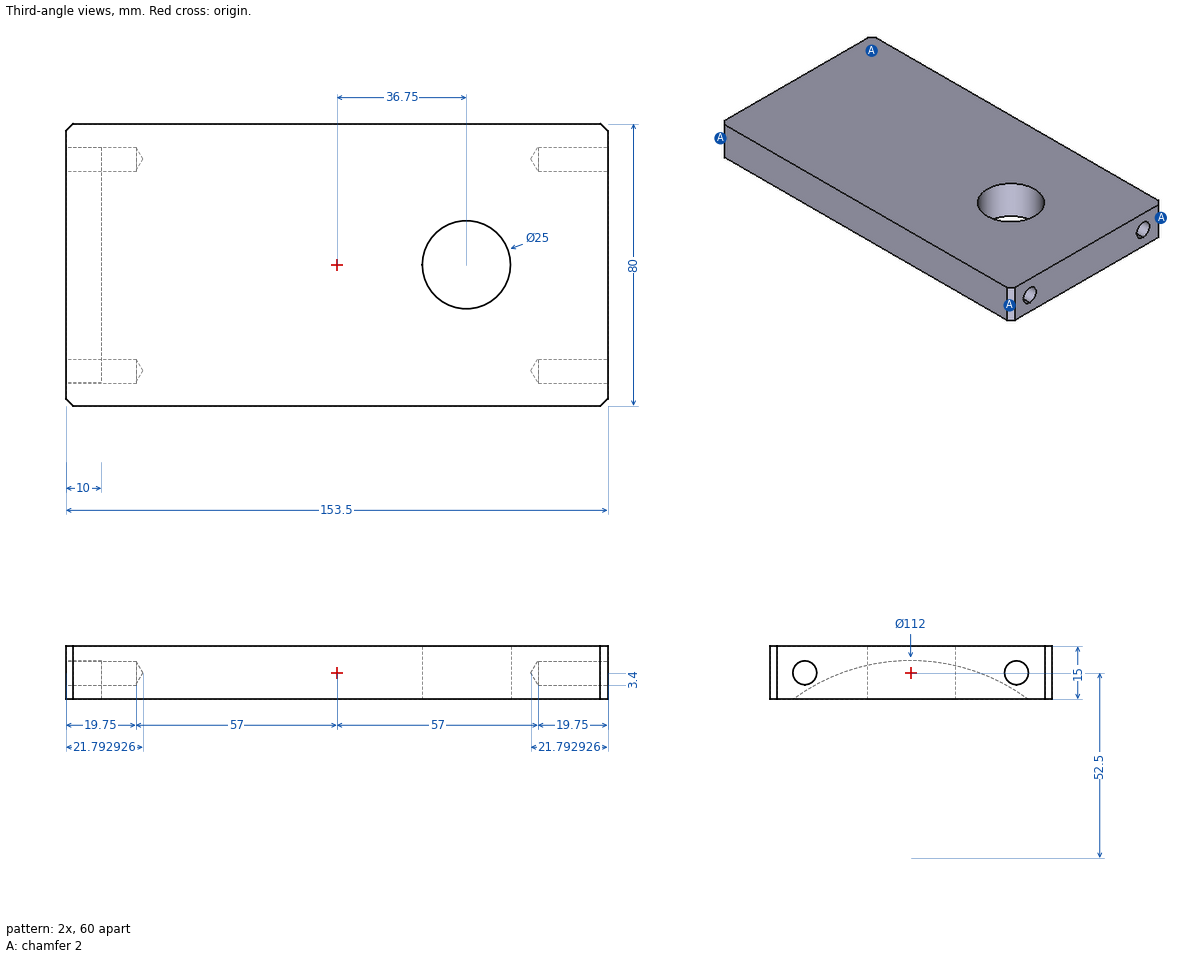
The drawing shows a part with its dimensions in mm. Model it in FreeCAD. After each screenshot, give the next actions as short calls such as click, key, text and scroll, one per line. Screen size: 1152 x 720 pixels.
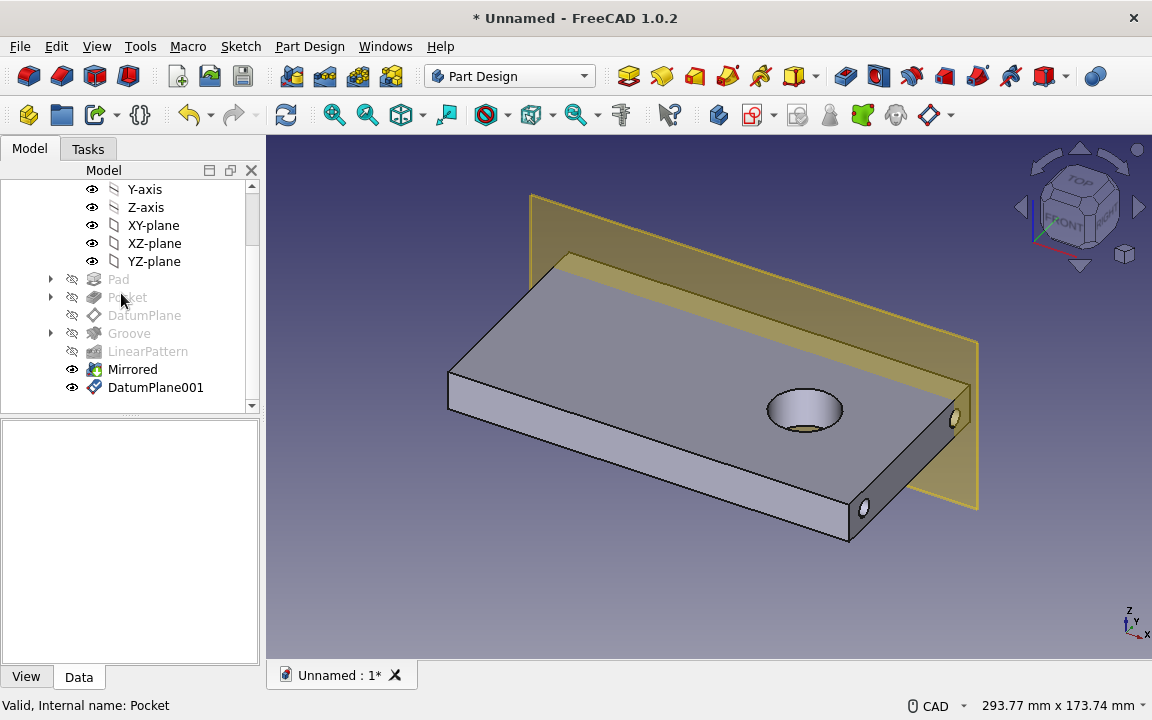
click(117, 387)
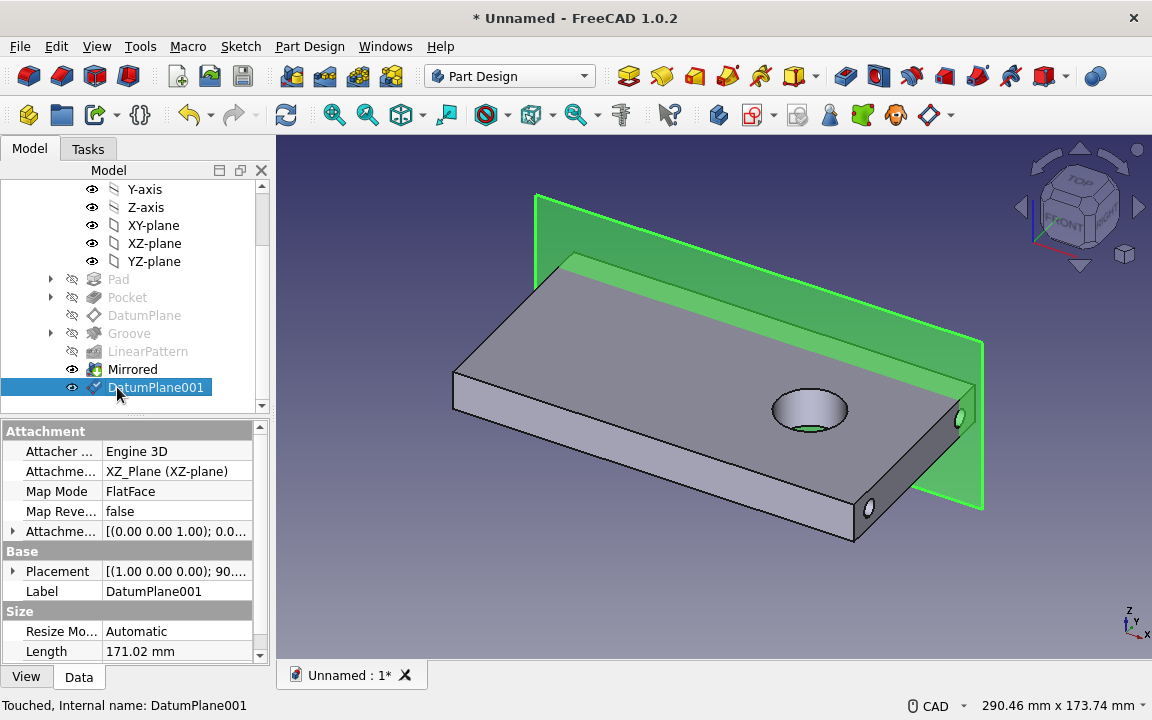
click(752, 116)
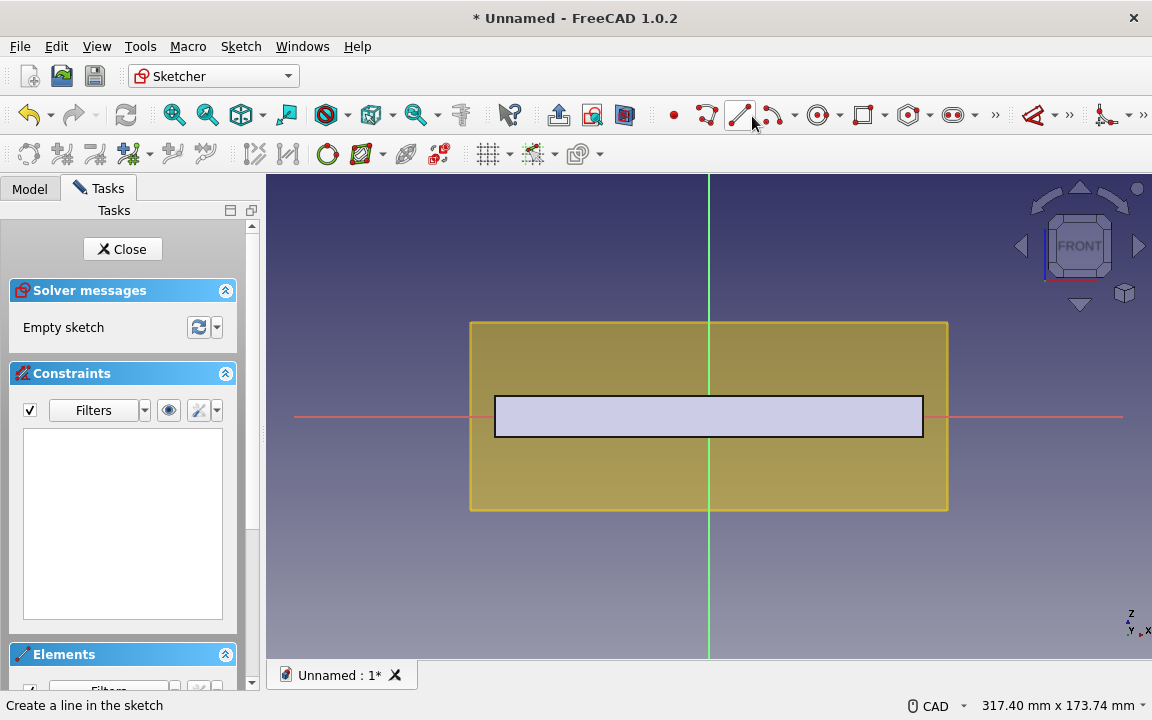
click(625, 116)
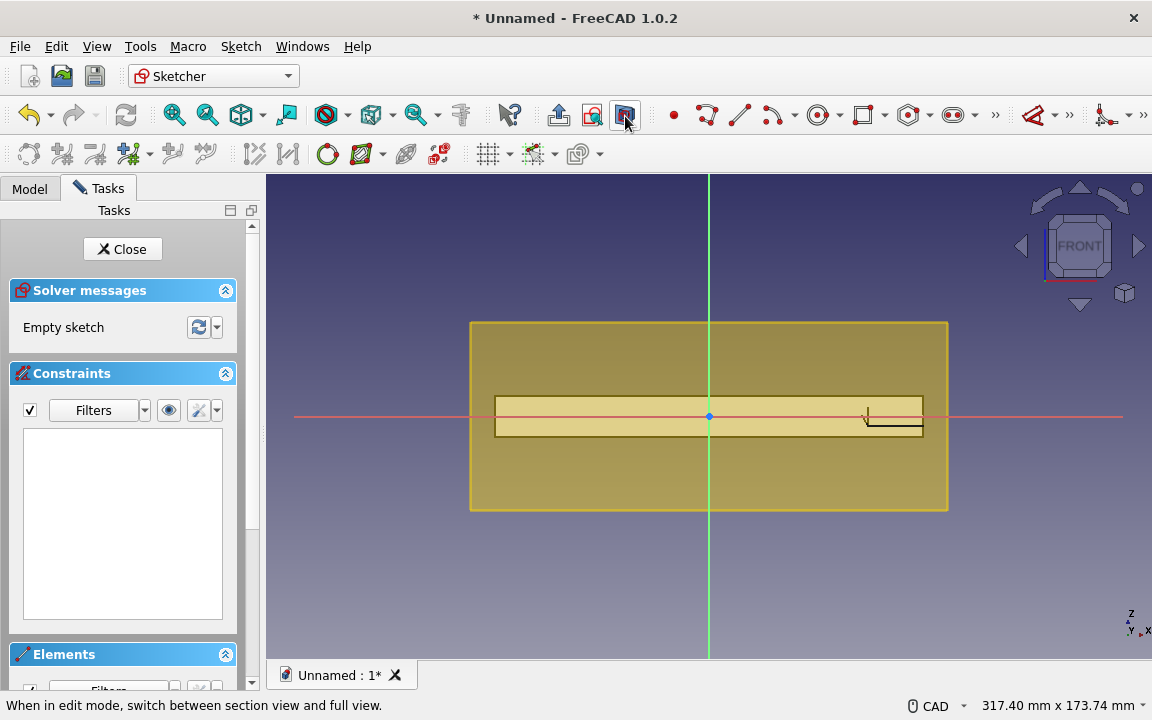
scroll(507, 422, up, 10)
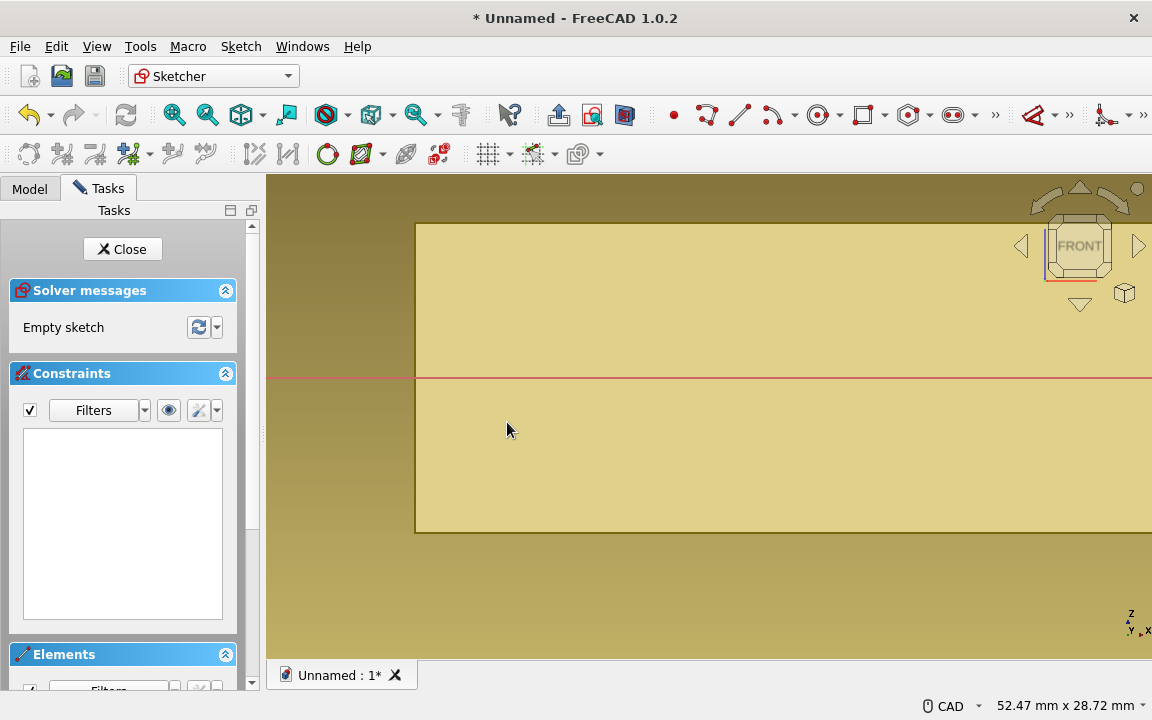
click(707, 116)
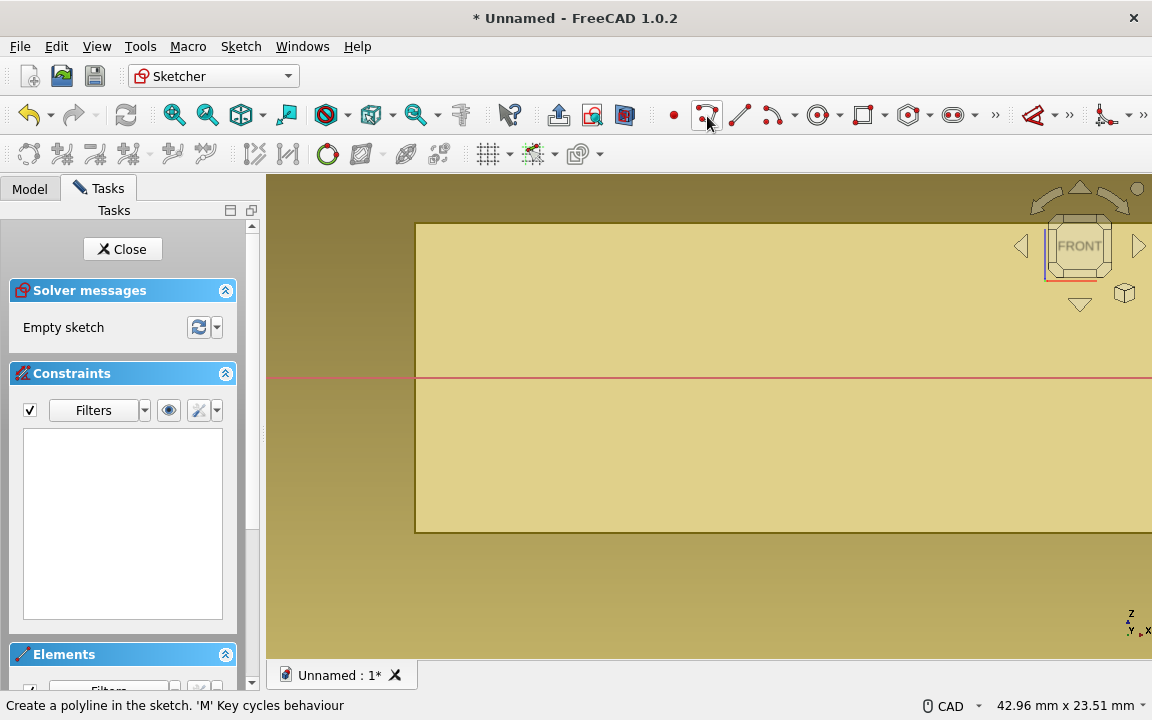
click(864, 378)
click(822, 448)
click(415, 448)
click(415, 387)
click(864, 378)
key(Escape)
key(Escape)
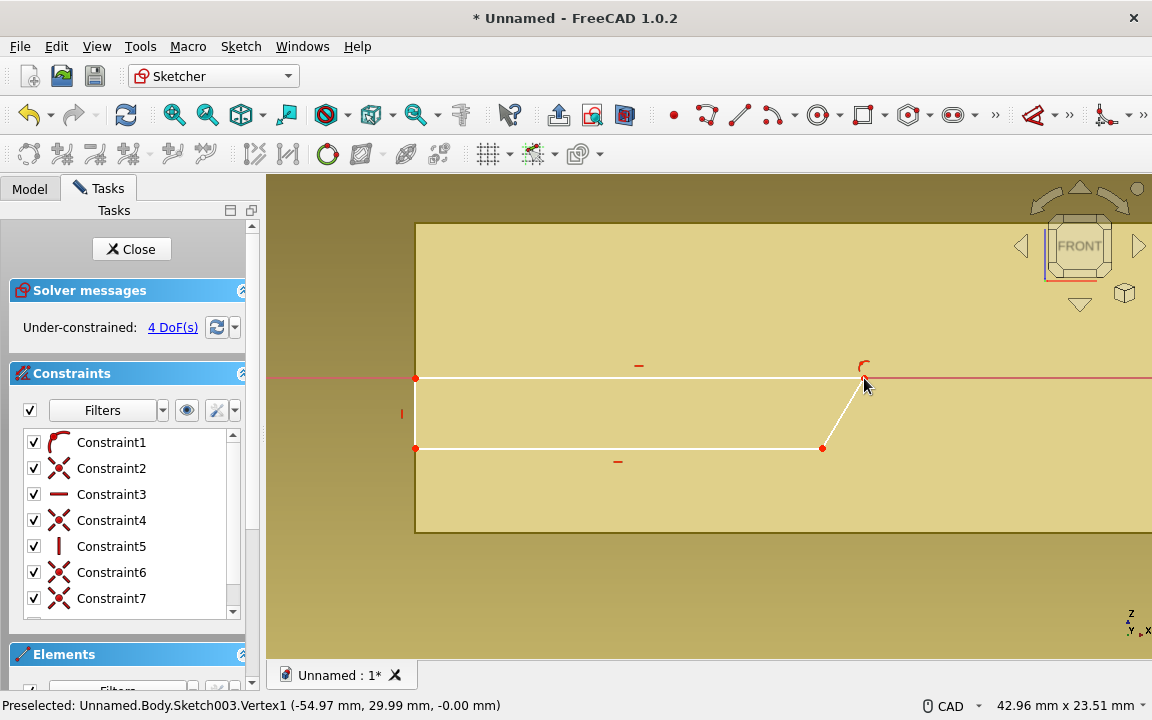
click(1032, 116)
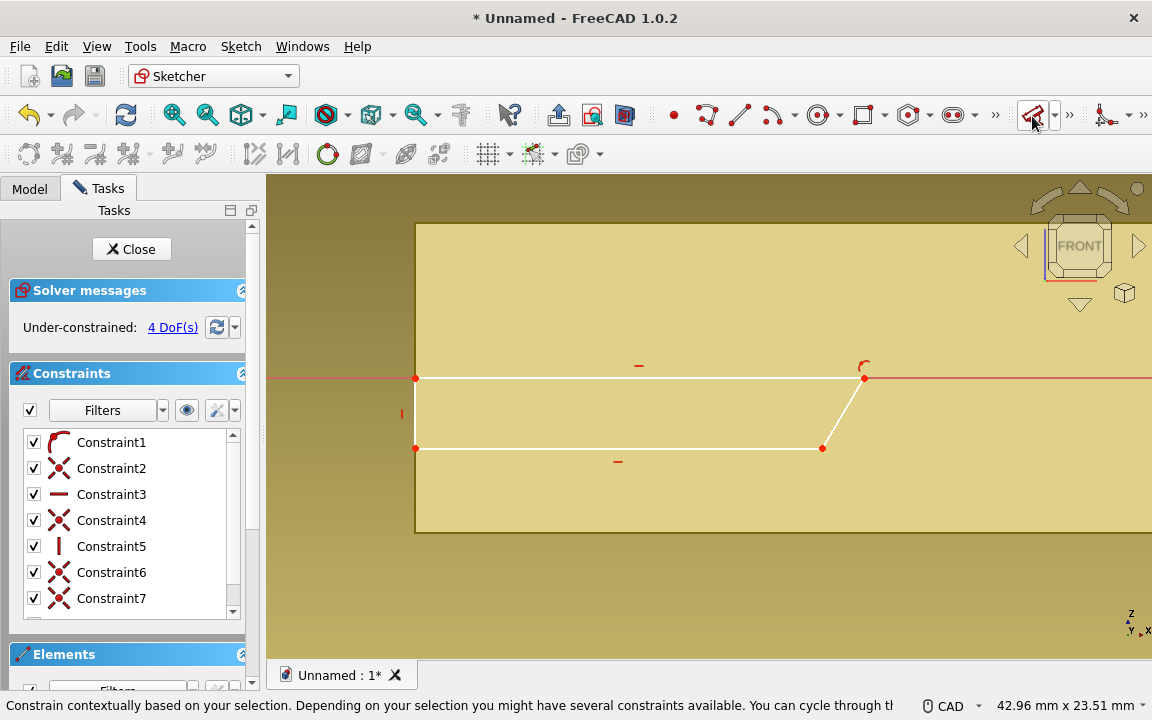
click(415, 428)
click(381, 414)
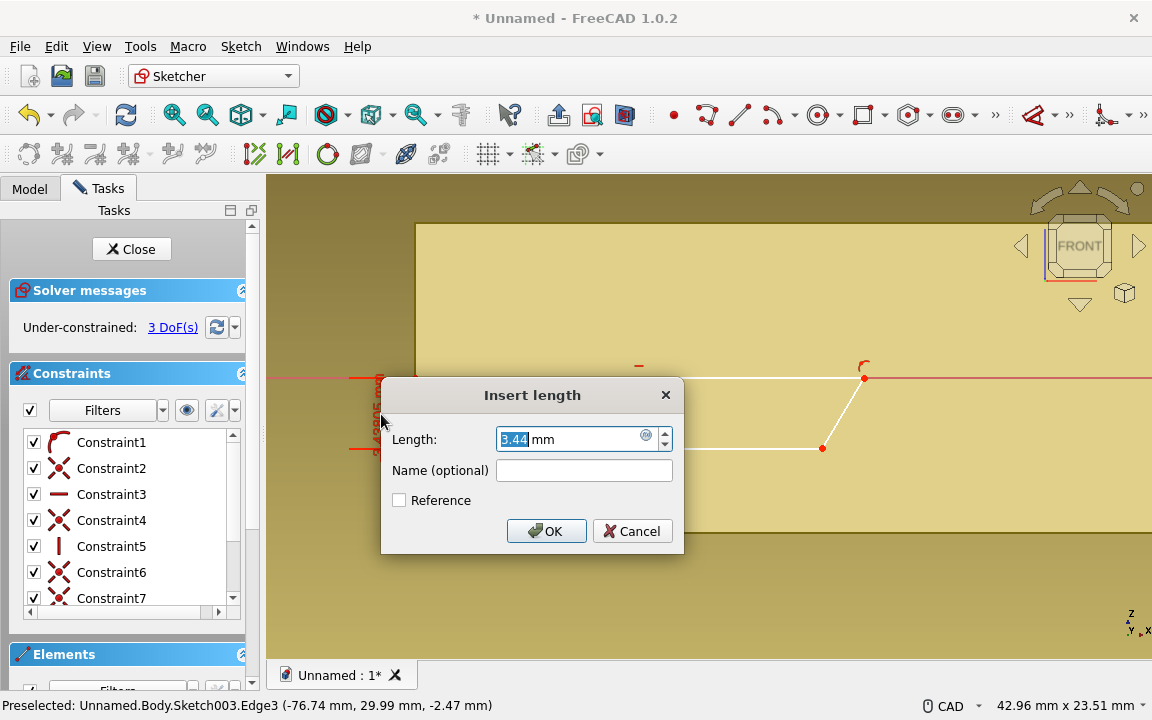
text(3.4)
key(Return)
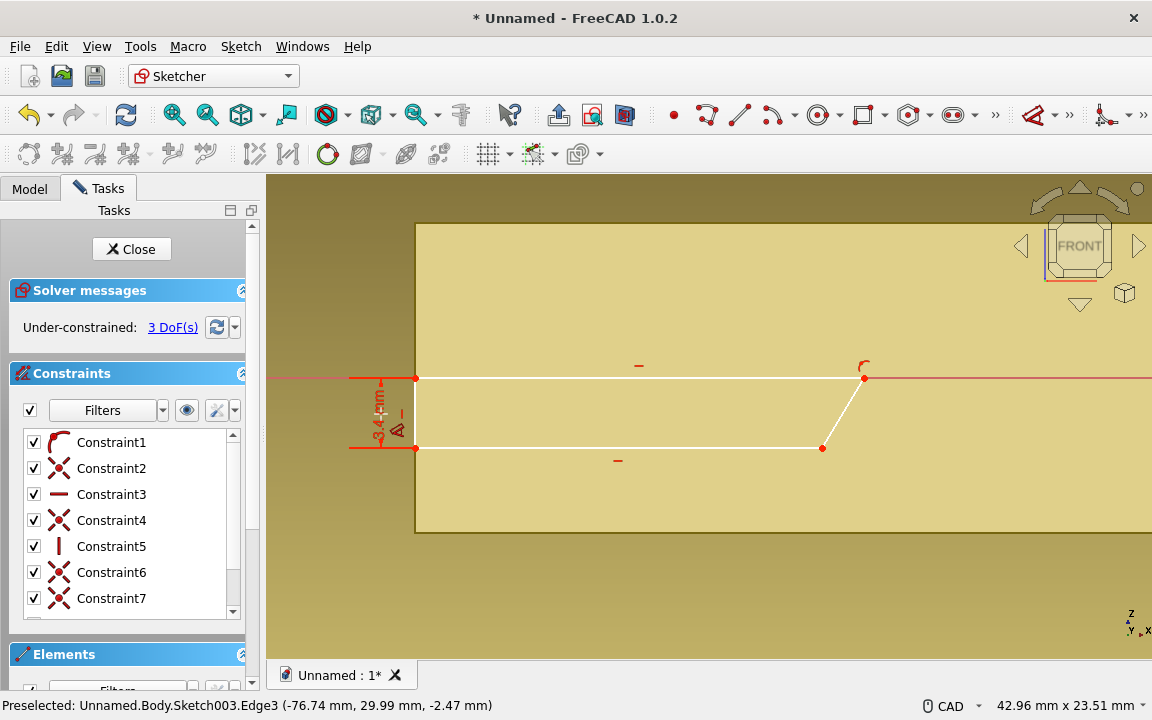
click(822, 448)
click(905, 482)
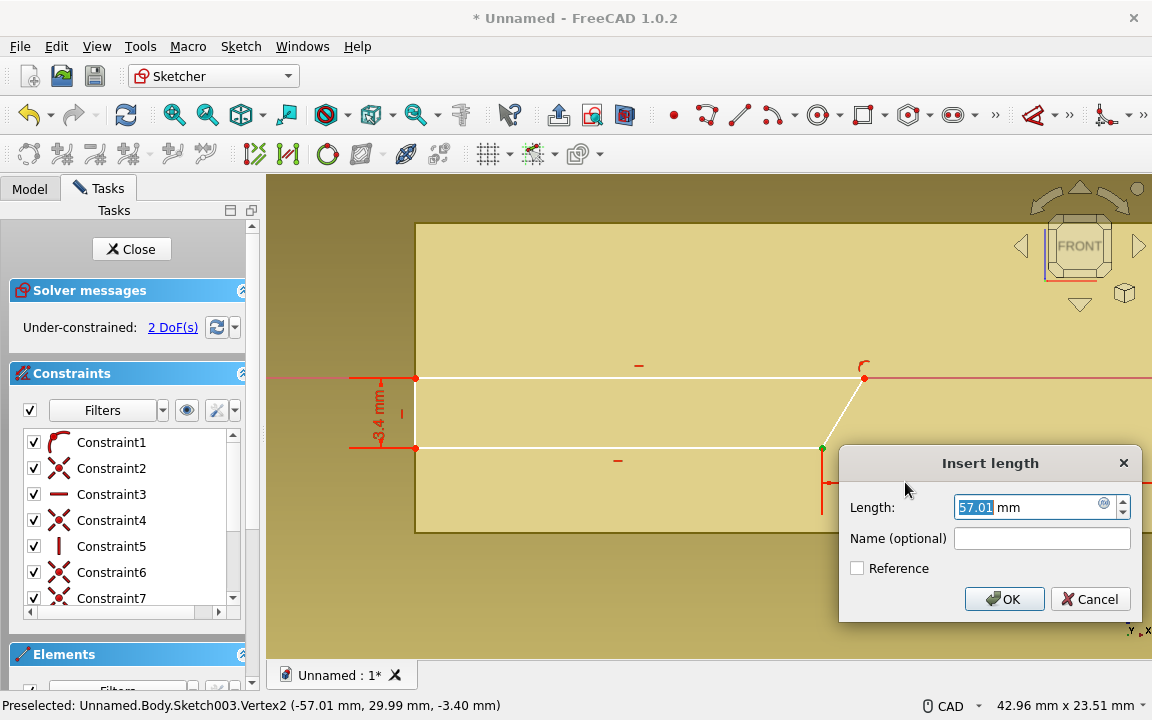
text(57)
key(Return)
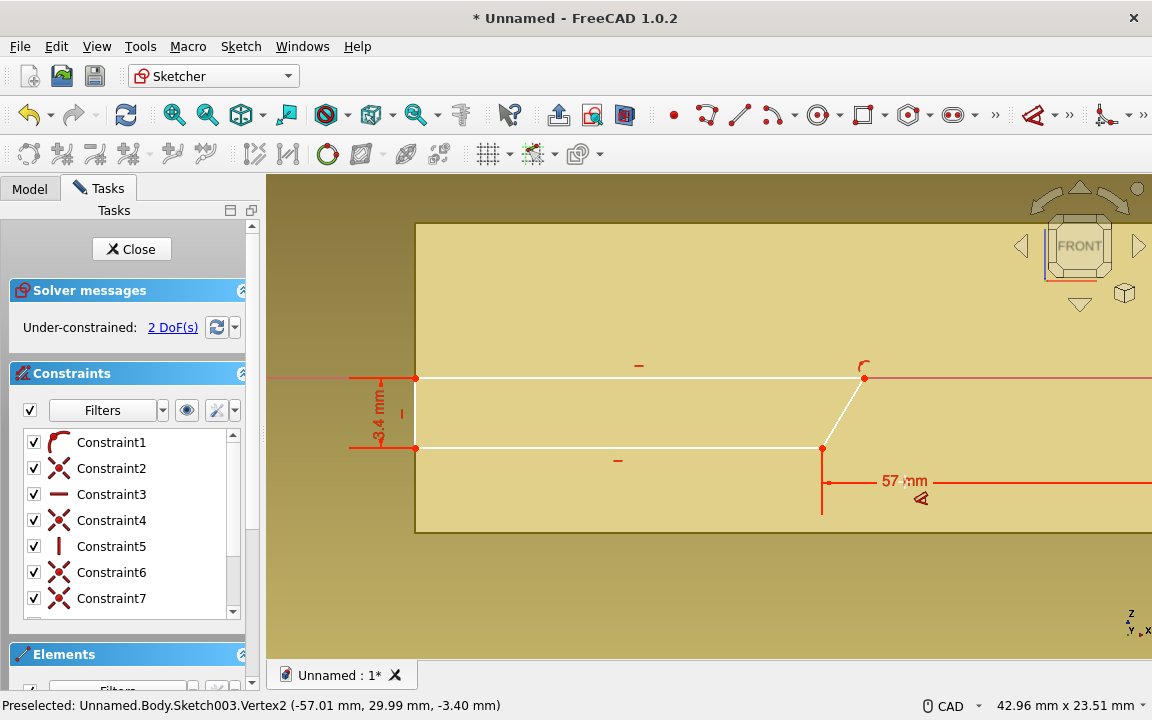
click(700, 448)
click(619, 482)